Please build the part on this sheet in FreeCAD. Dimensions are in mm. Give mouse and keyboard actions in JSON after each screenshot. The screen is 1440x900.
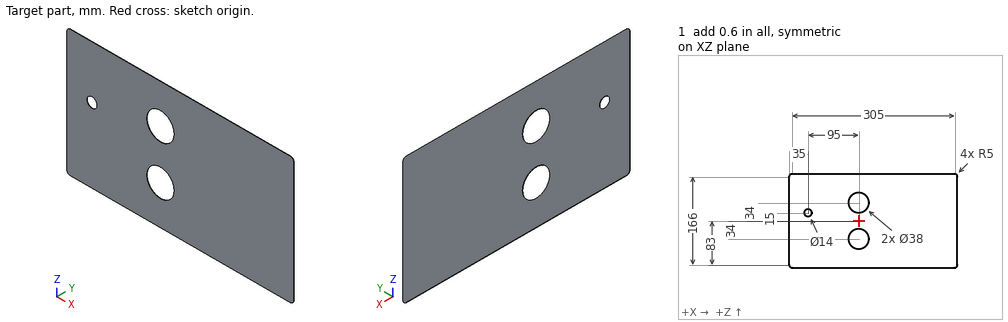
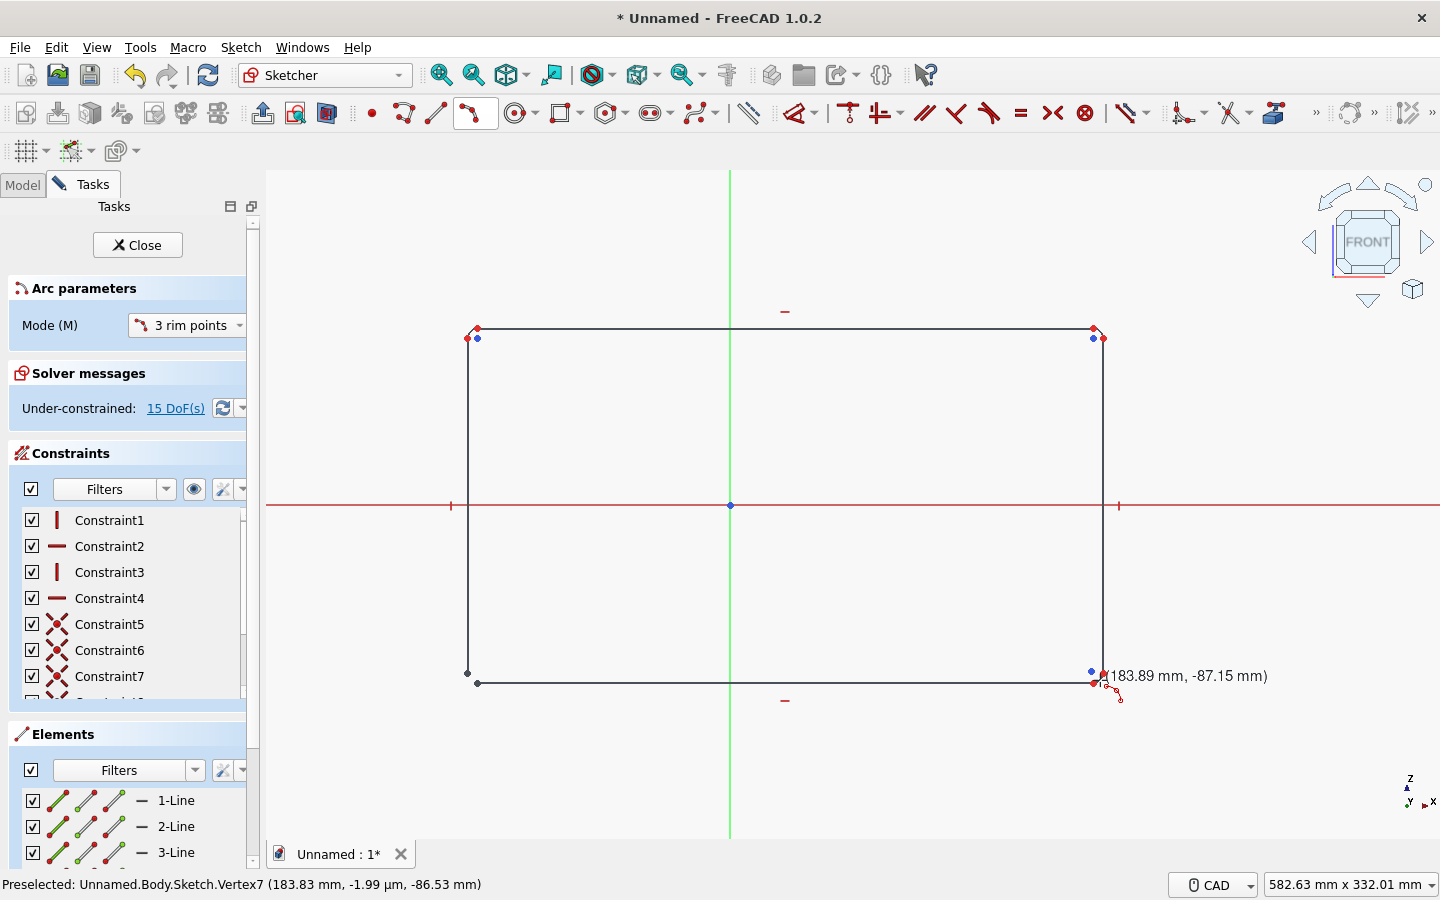
{"action": "left_click", "coordinate": [478, 683]}
{"action": "left_click", "coordinate": [468, 673]}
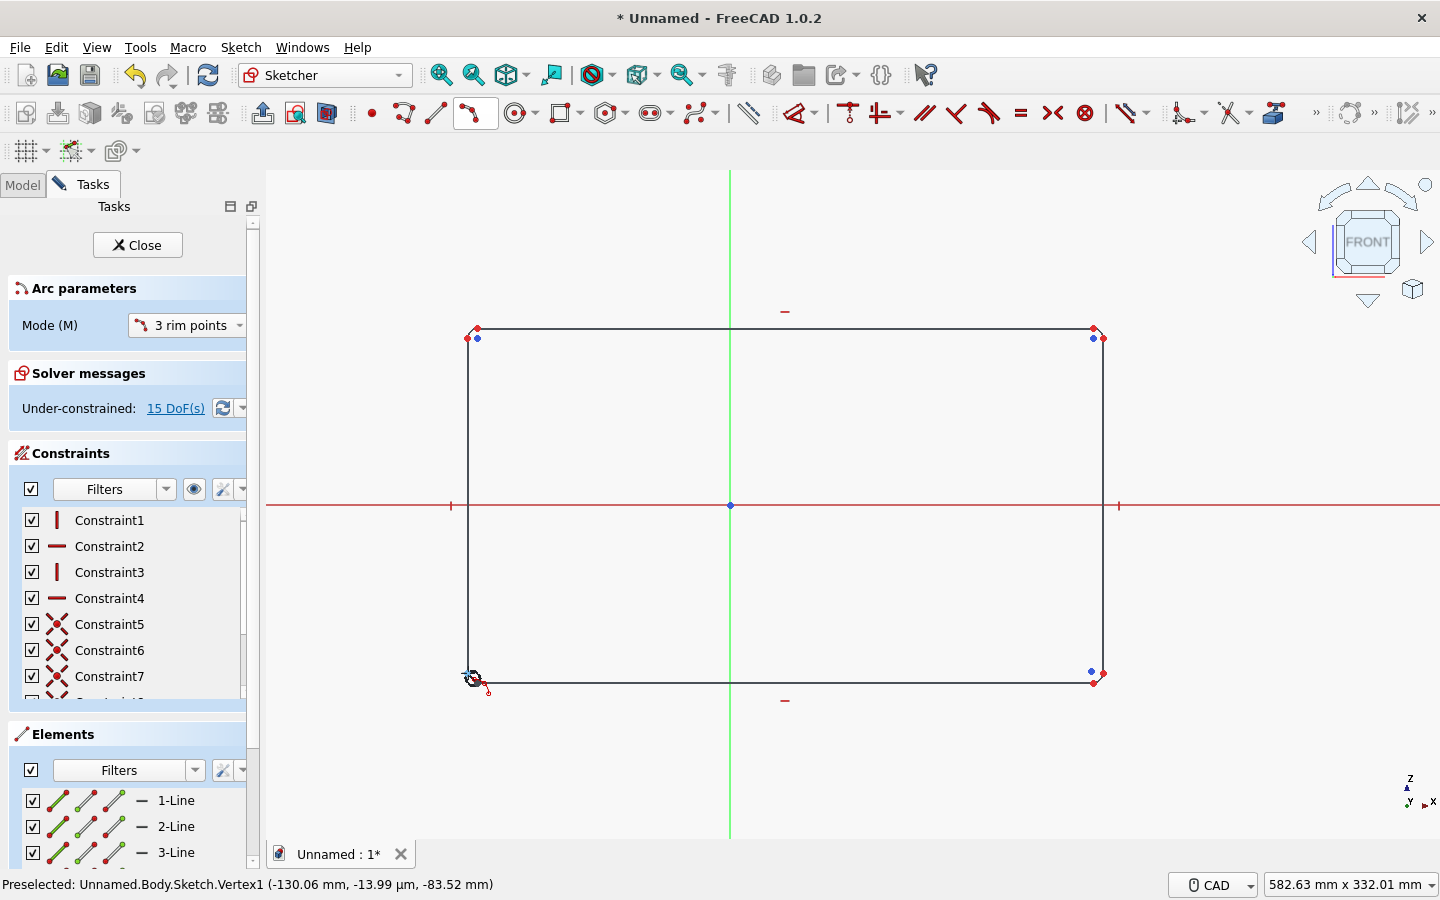
{"action": "scroll", "coordinate": [471, 680], "scroll_direction": "up", "scroll_amount": 9}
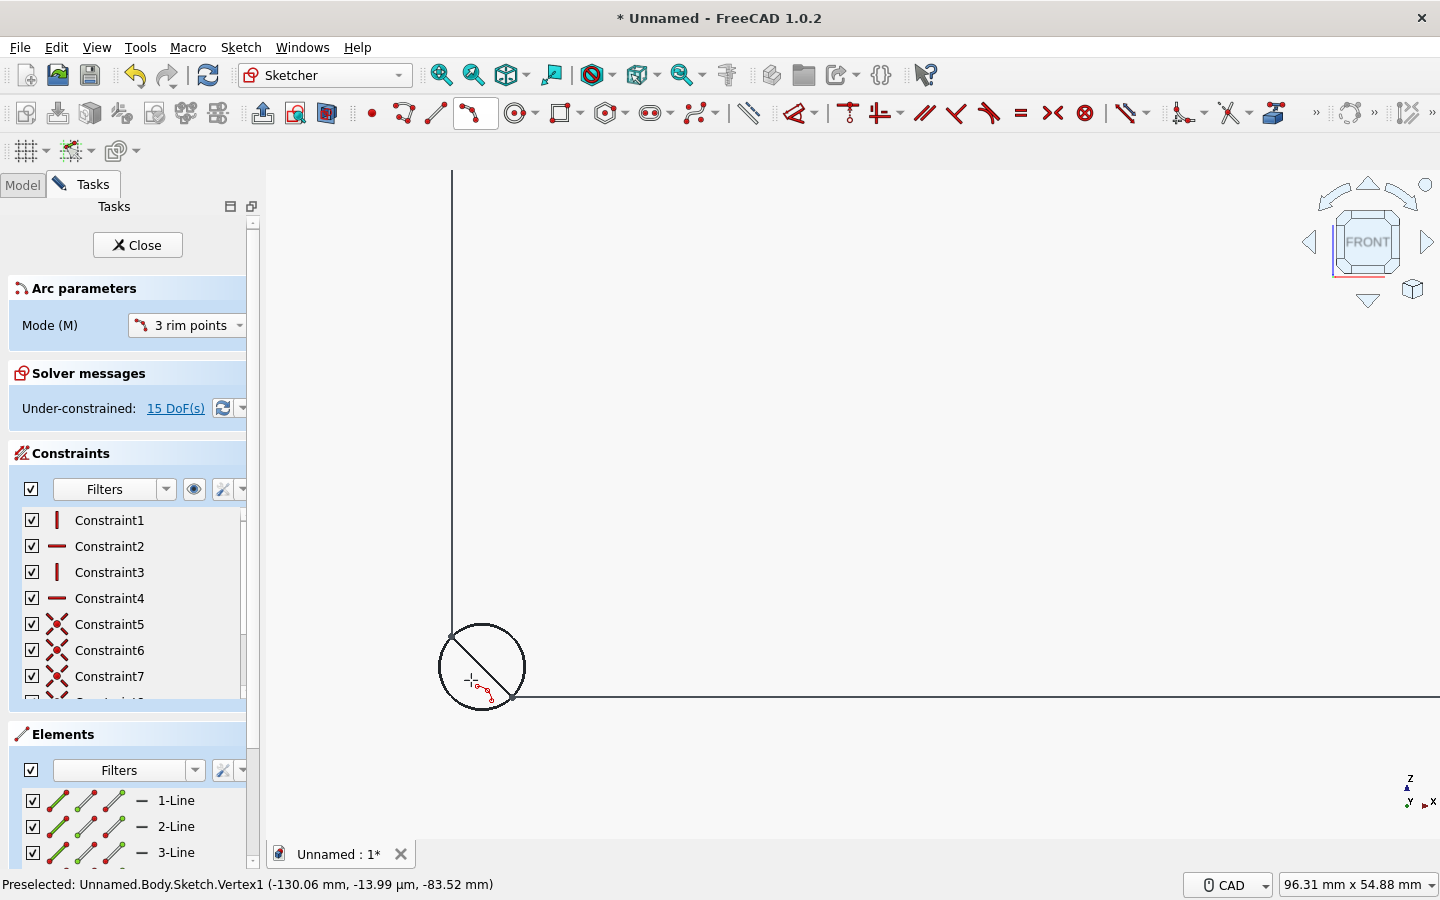
{"action": "left_click", "coordinate": [471, 674]}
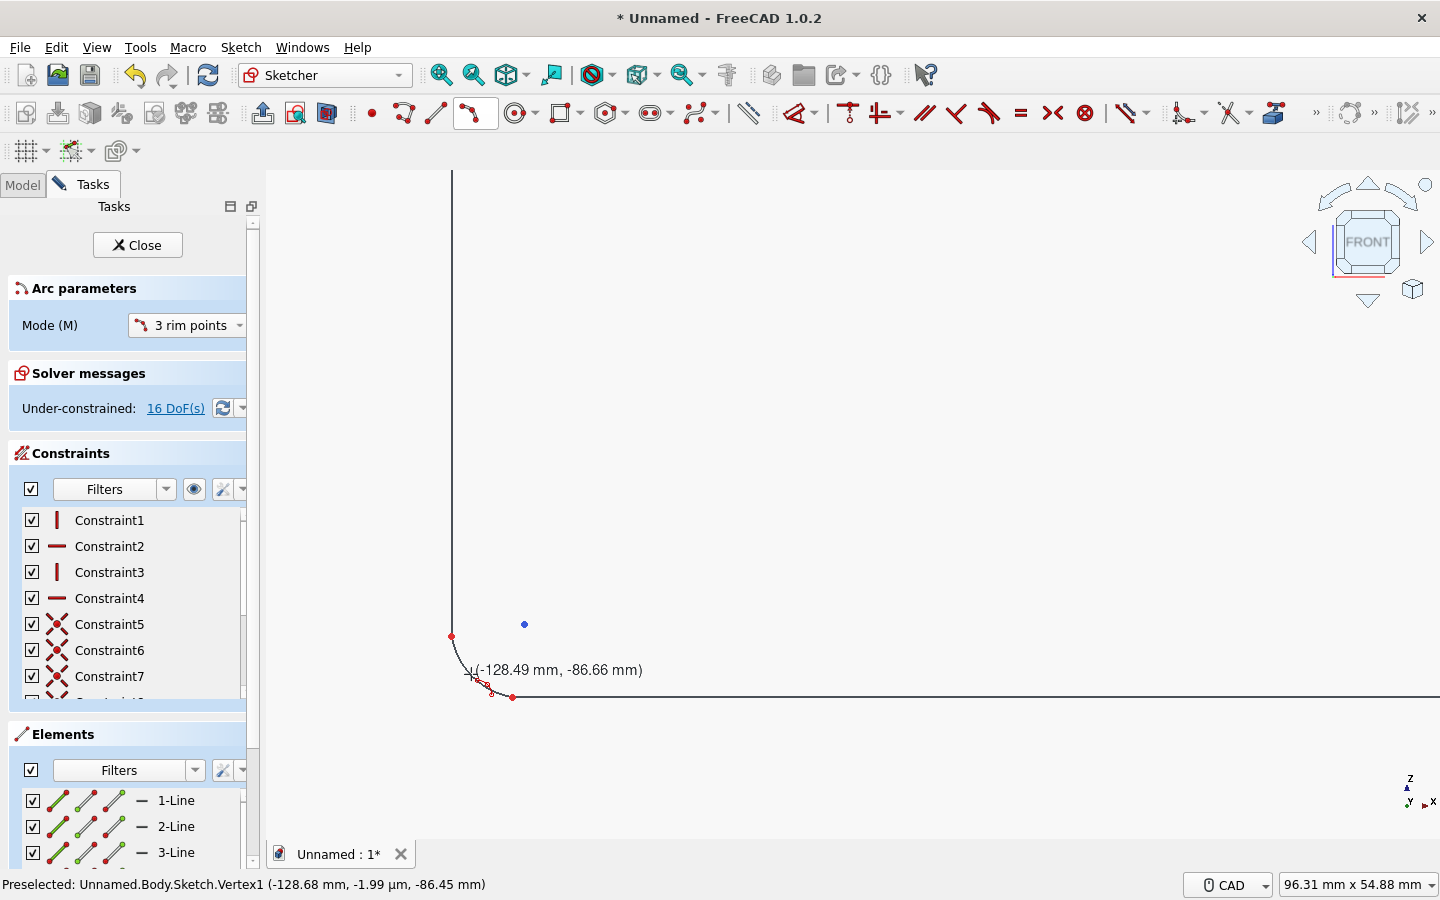
{"action": "left_click", "coordinate": [516, 114]}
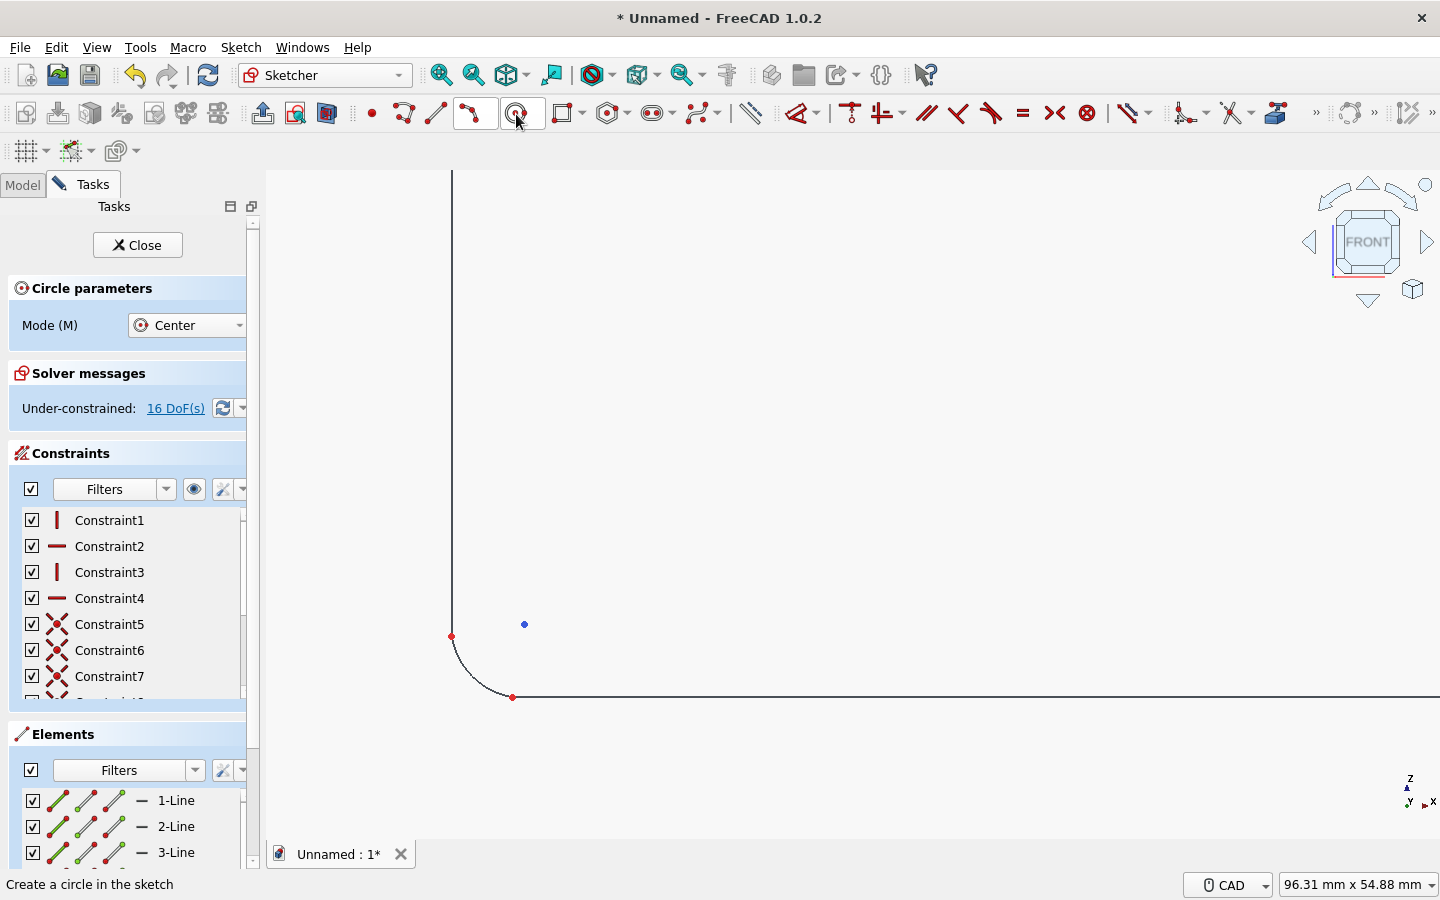
{"action": "scroll", "coordinate": [470, 680], "scroll_direction": "down", "scroll_amount": 9}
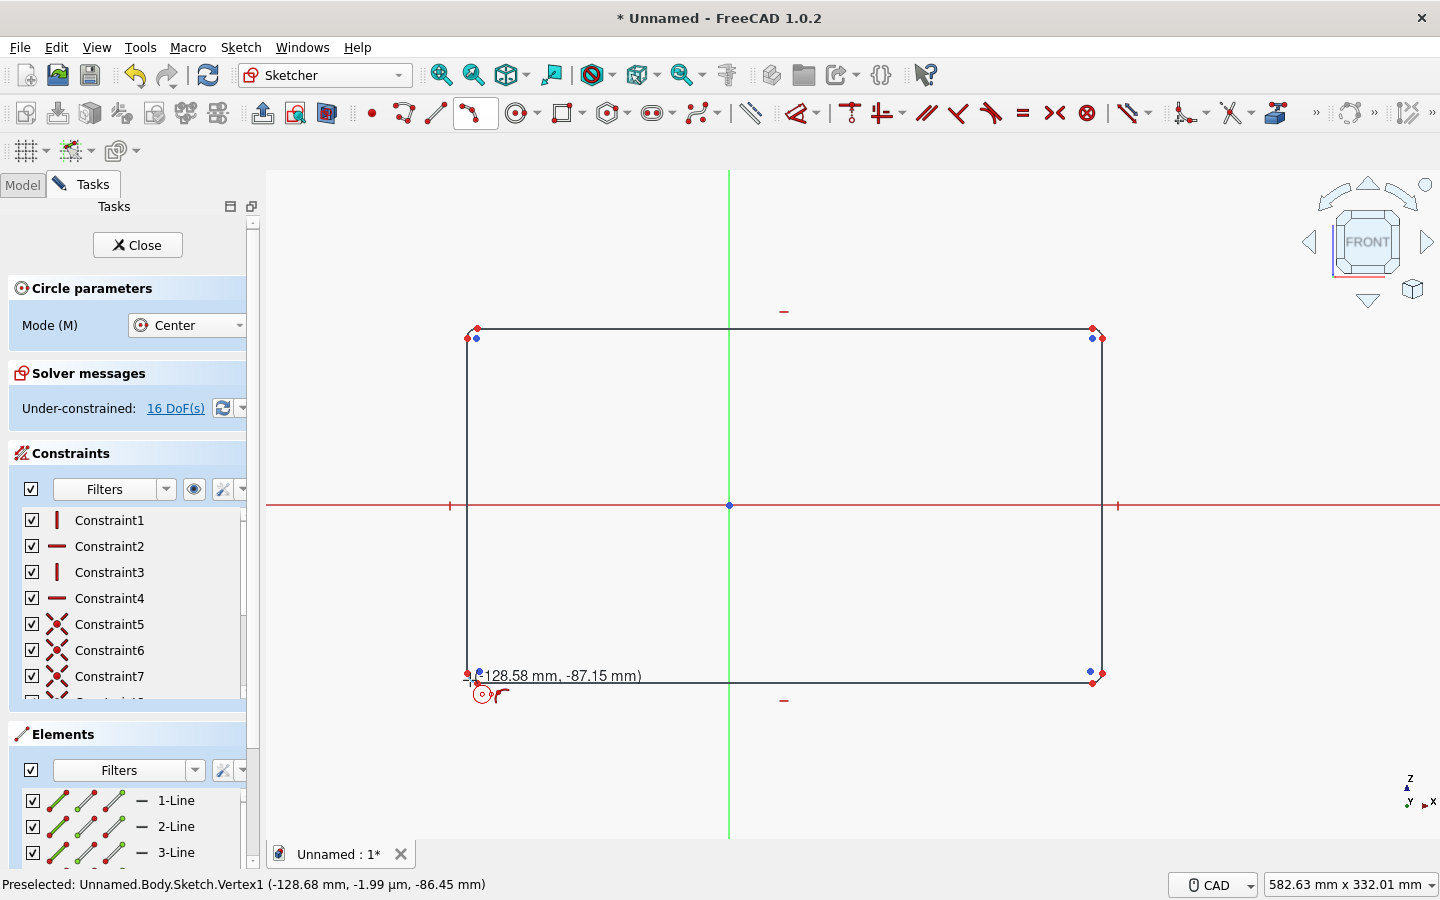
{"action": "scroll", "coordinate": [538, 475], "scroll_direction": "up", "scroll_amount": 3}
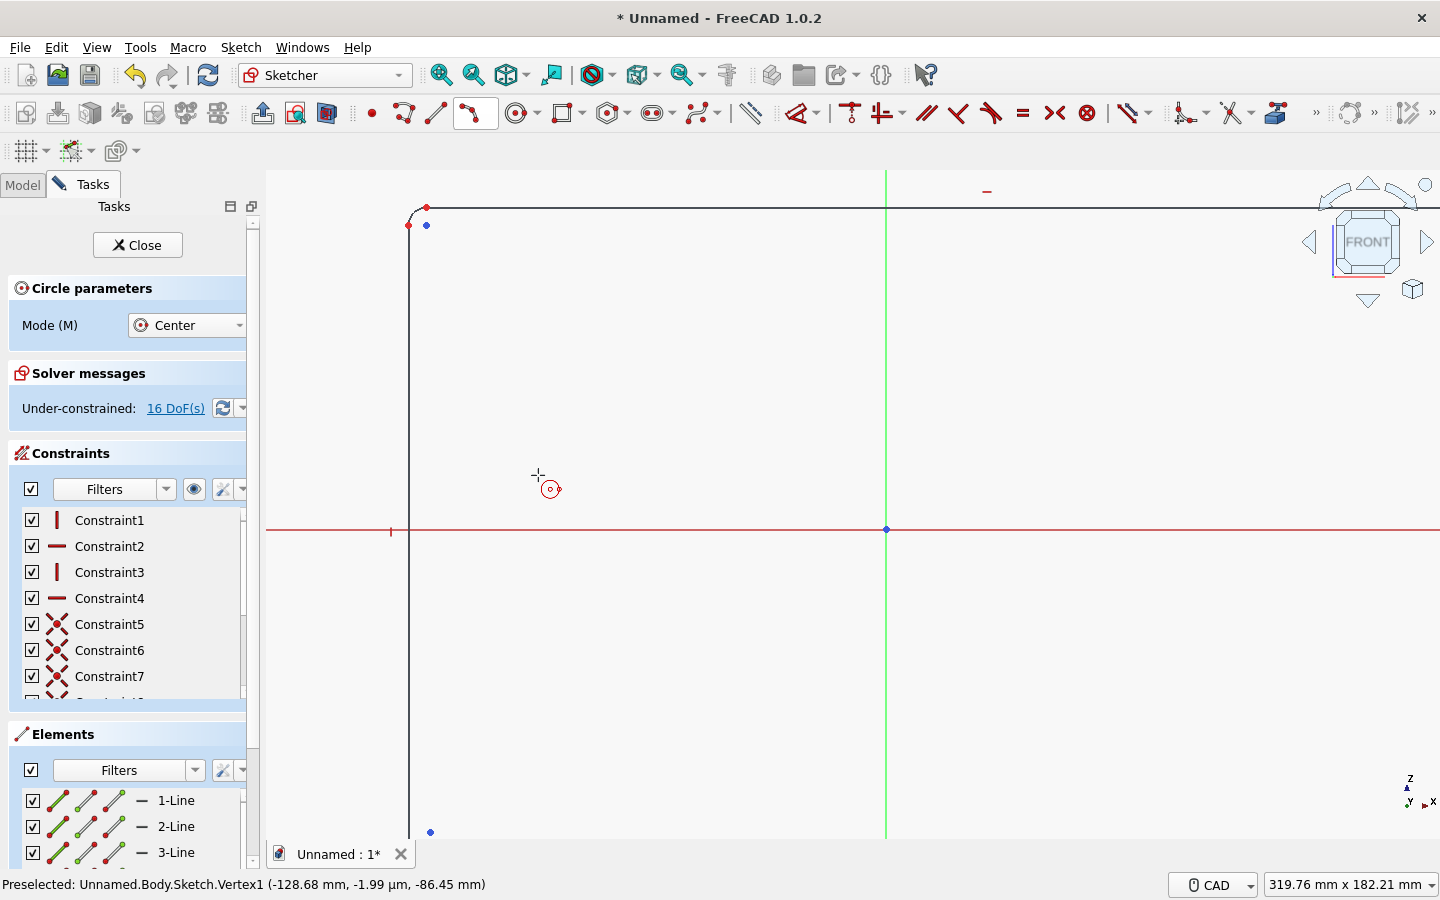
{"action": "left_click", "coordinate": [537, 475]}
{"action": "mouse_move", "coordinate": [556, 456]}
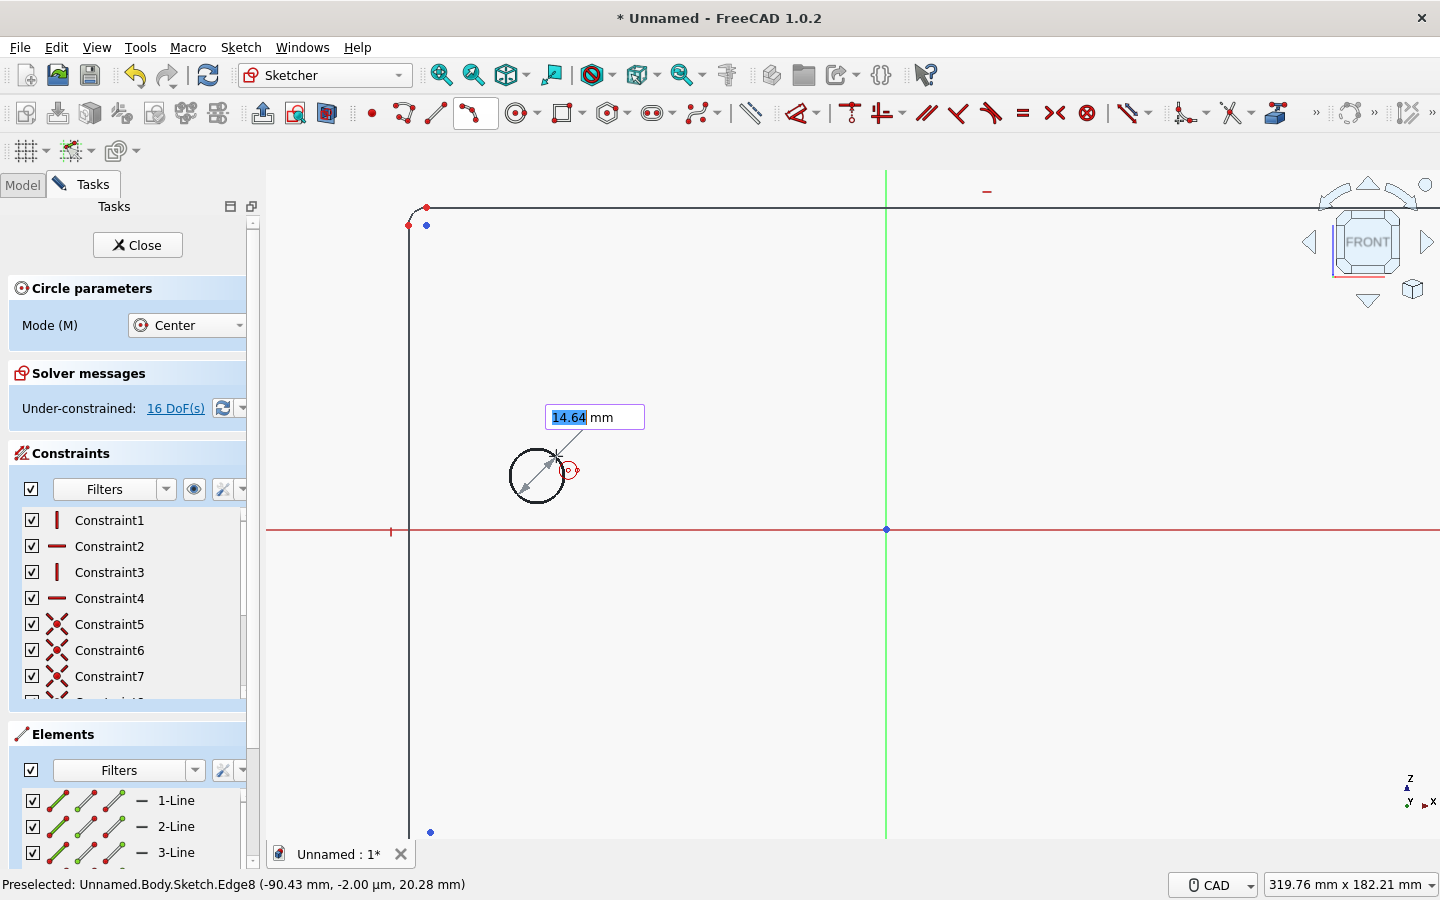
{"action": "type", "text": "14"}
{"action": "key", "text": "Return"}